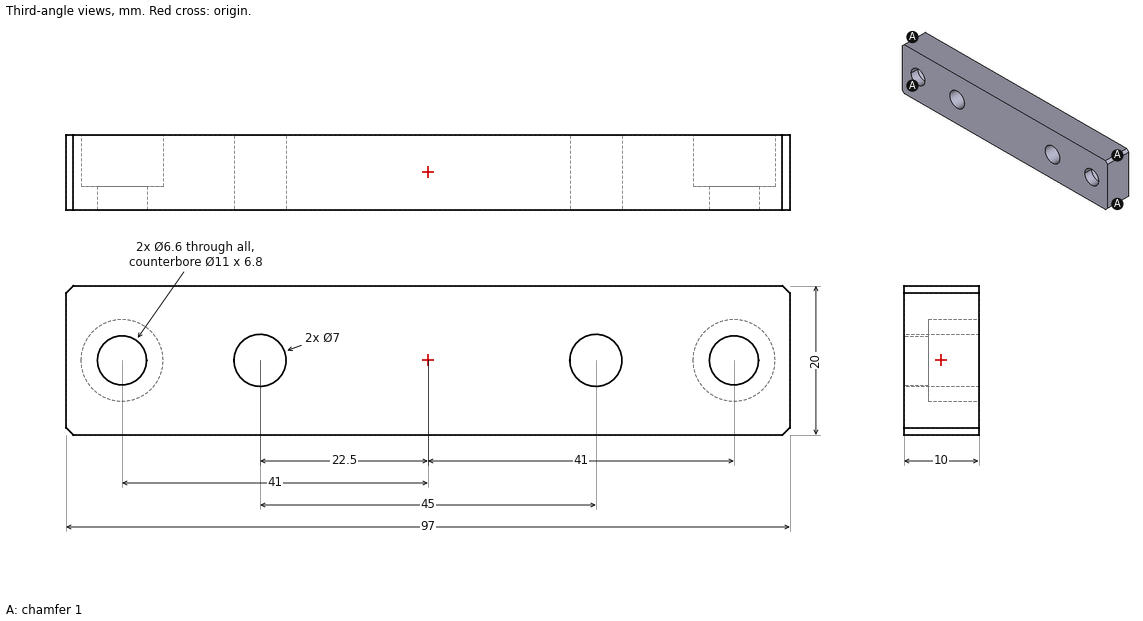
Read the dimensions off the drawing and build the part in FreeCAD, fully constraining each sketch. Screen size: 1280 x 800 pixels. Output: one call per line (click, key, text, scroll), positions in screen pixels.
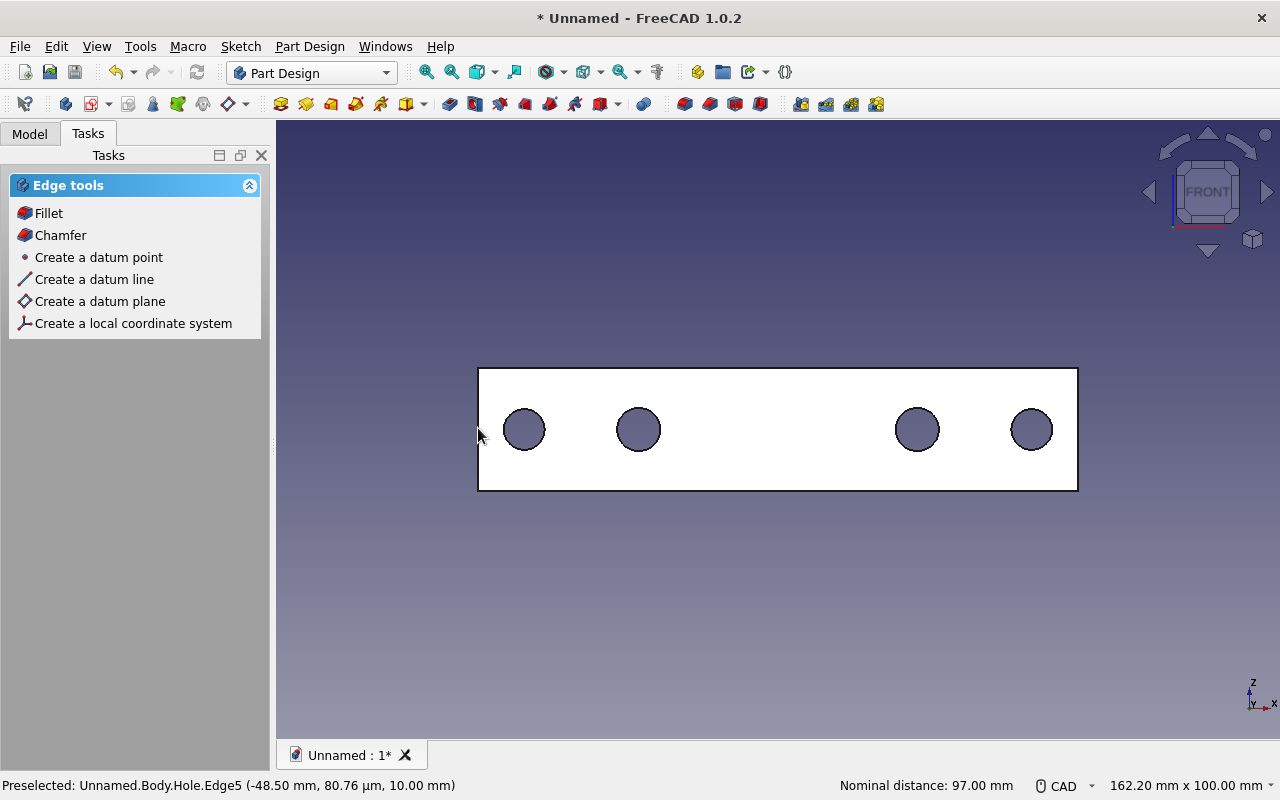
key(3)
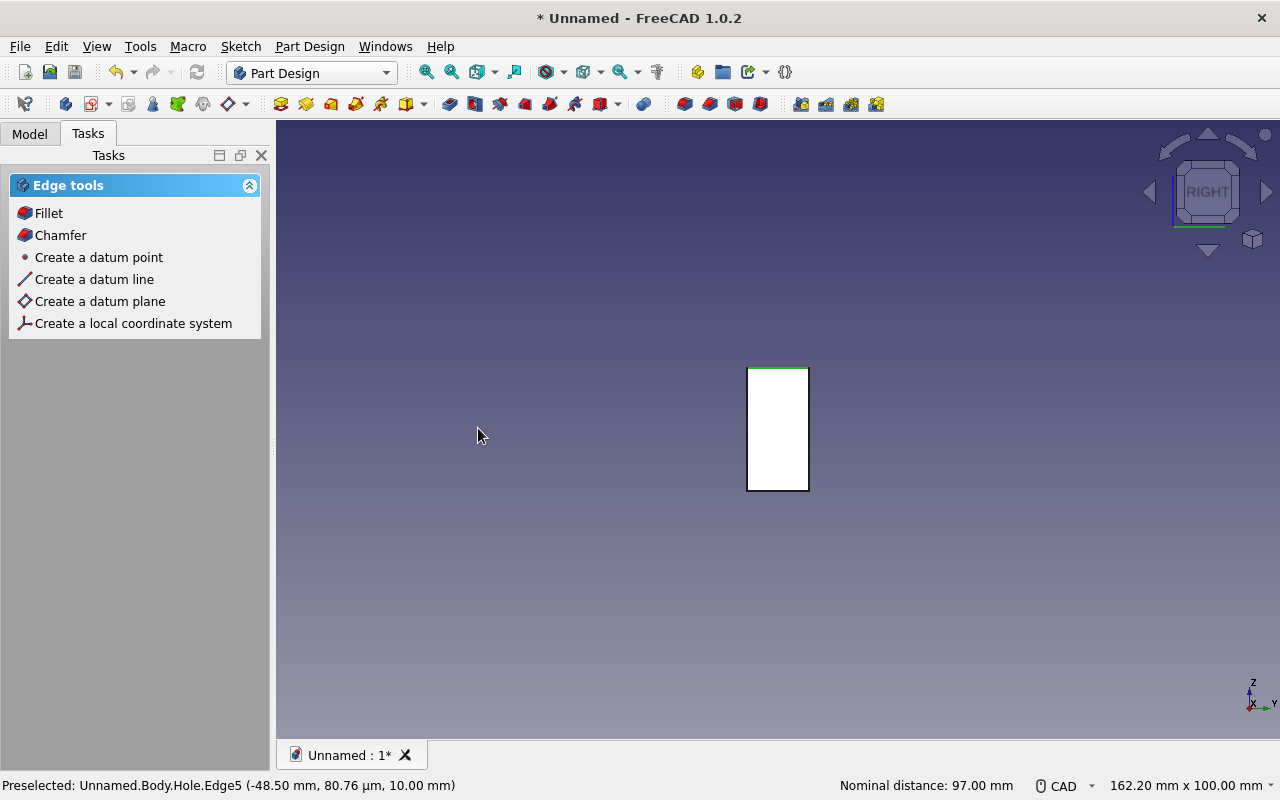
key(v)
key(f)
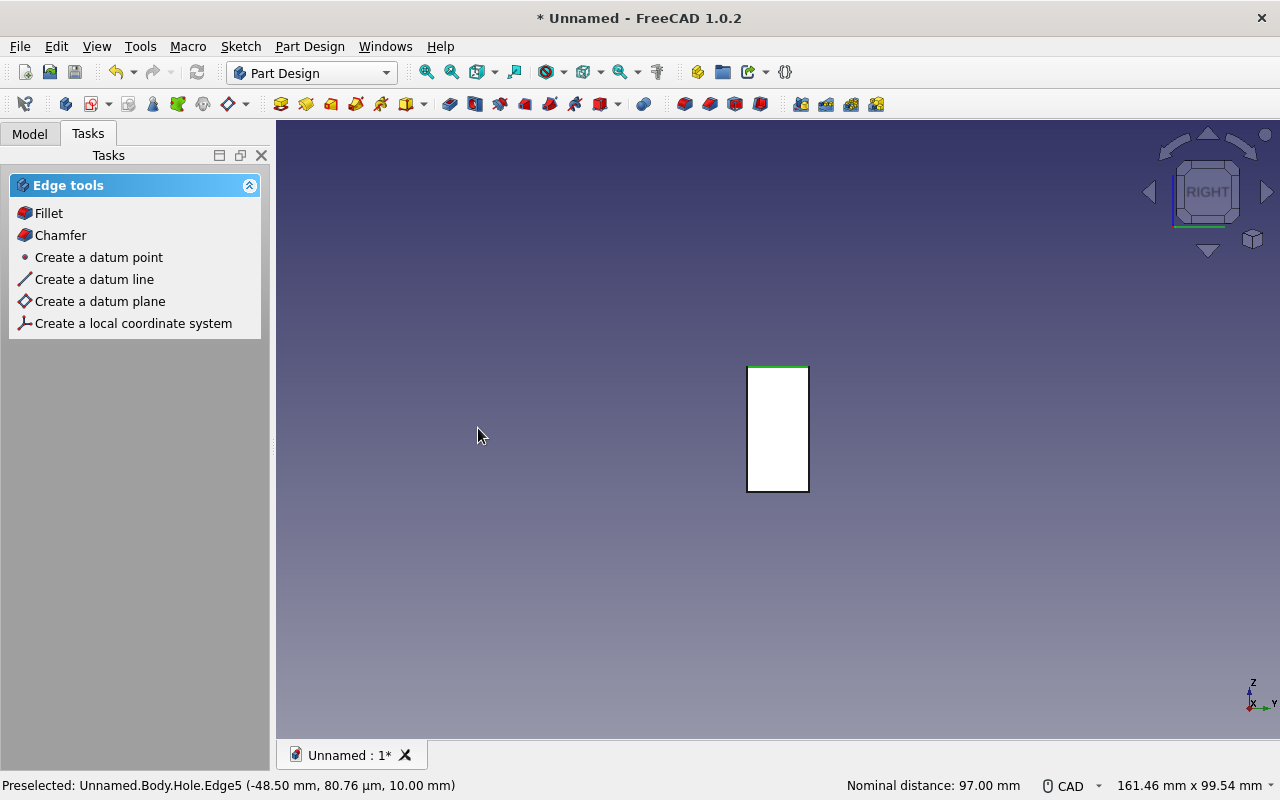
click(778, 491, ctrl)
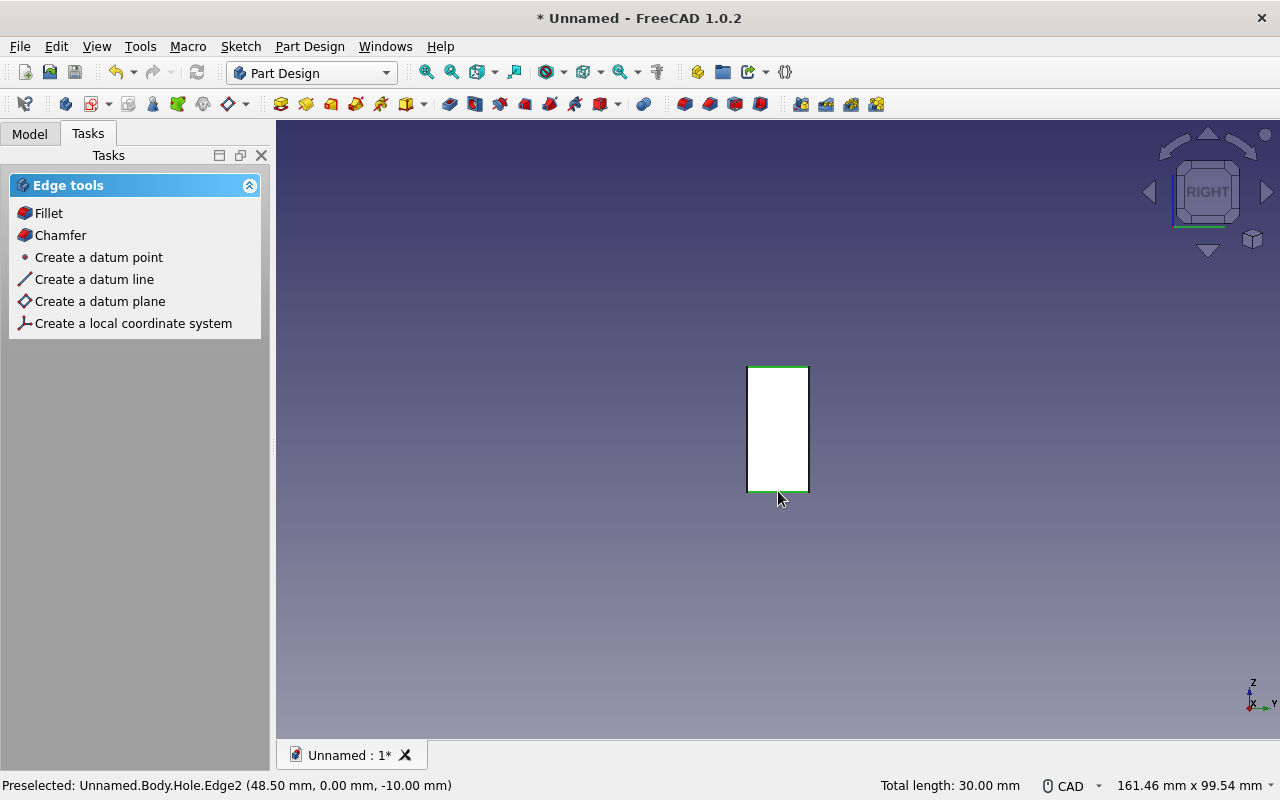
key(5)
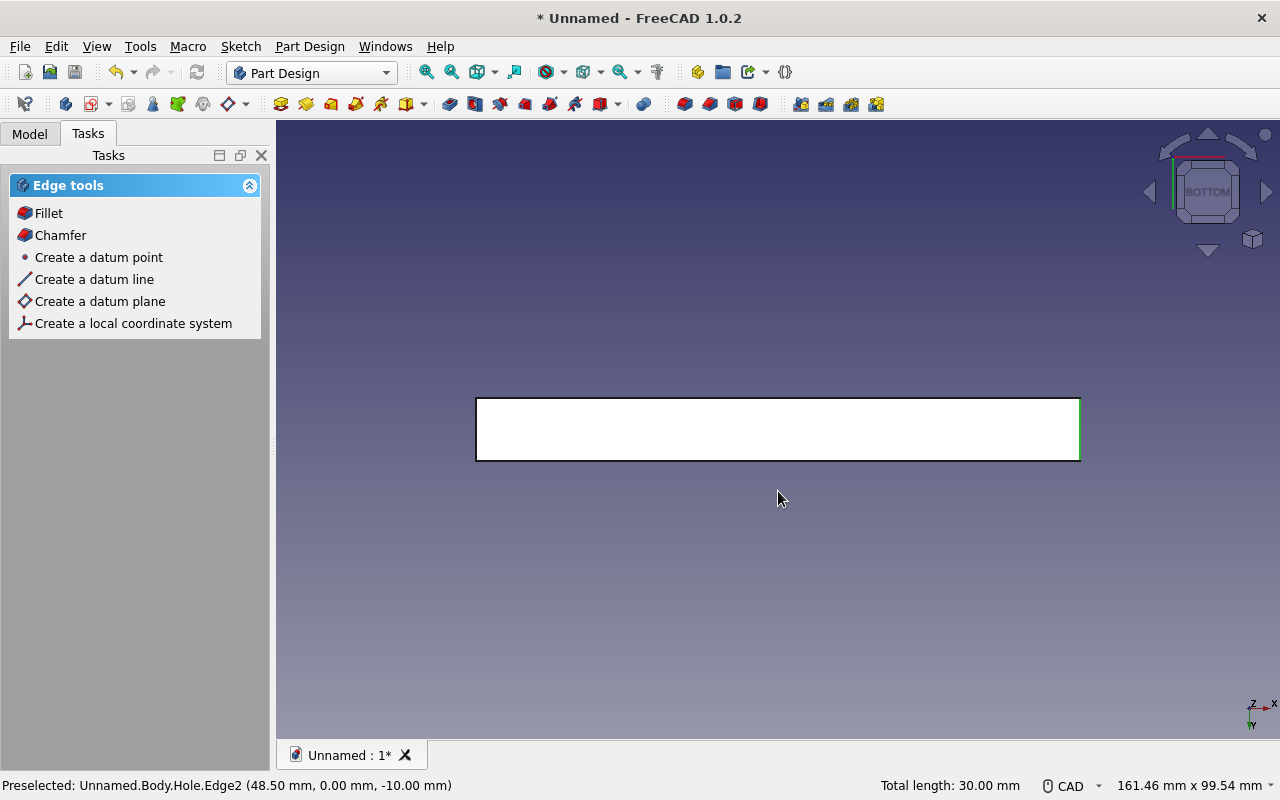
click(476, 428, ctrl)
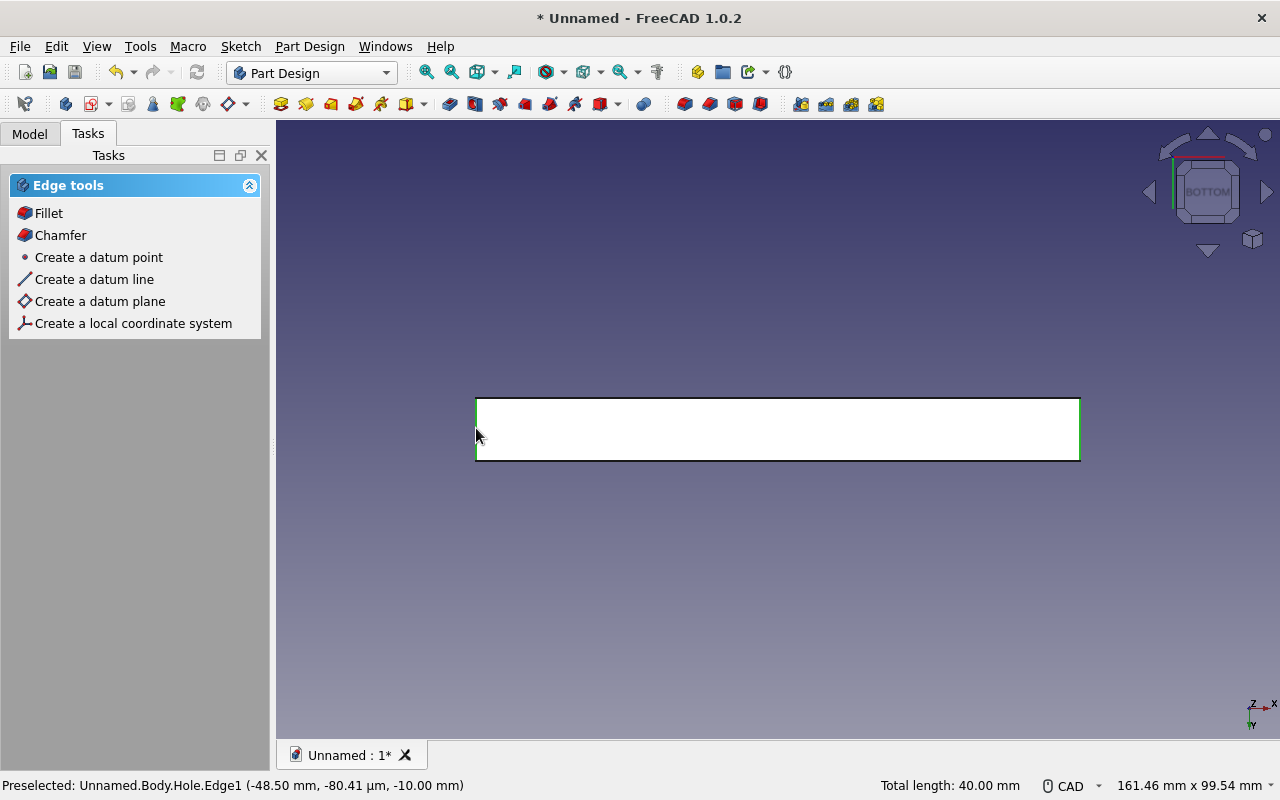
click(710, 104)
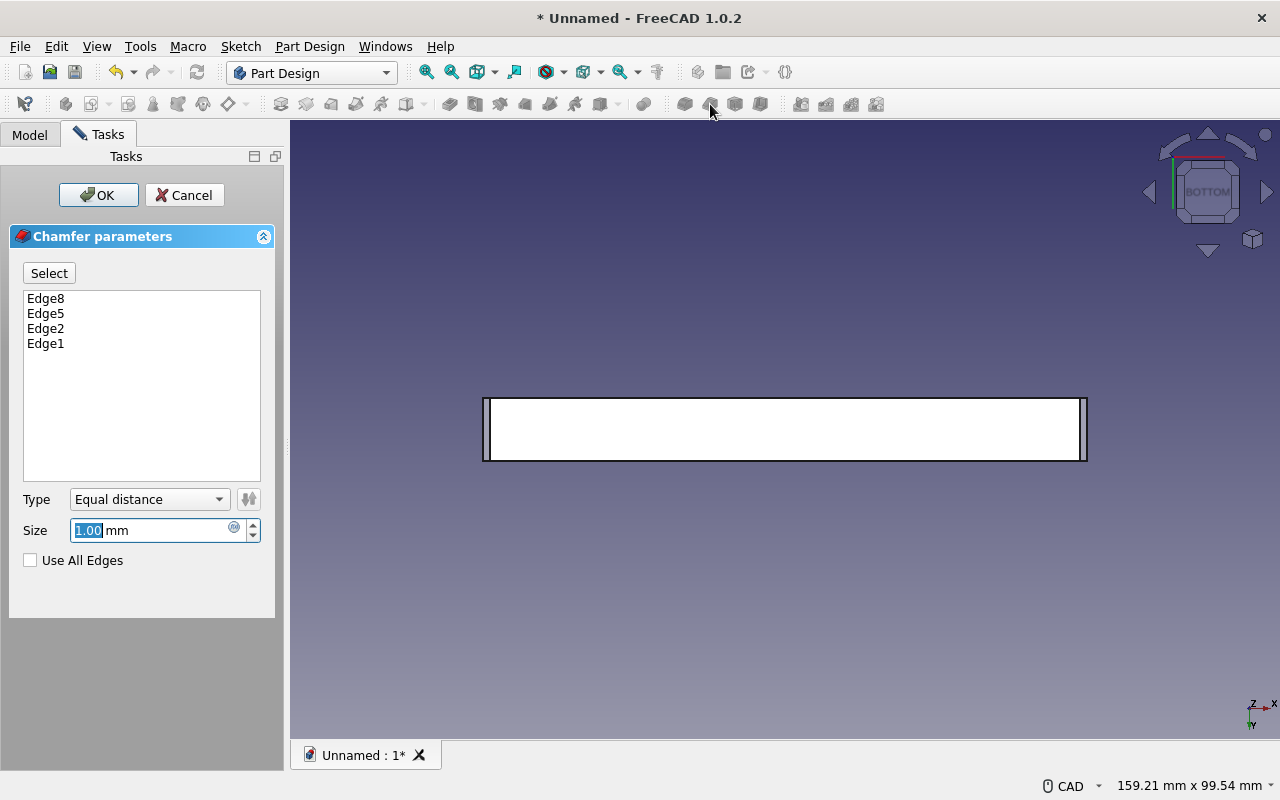
text(1)
key(Tab)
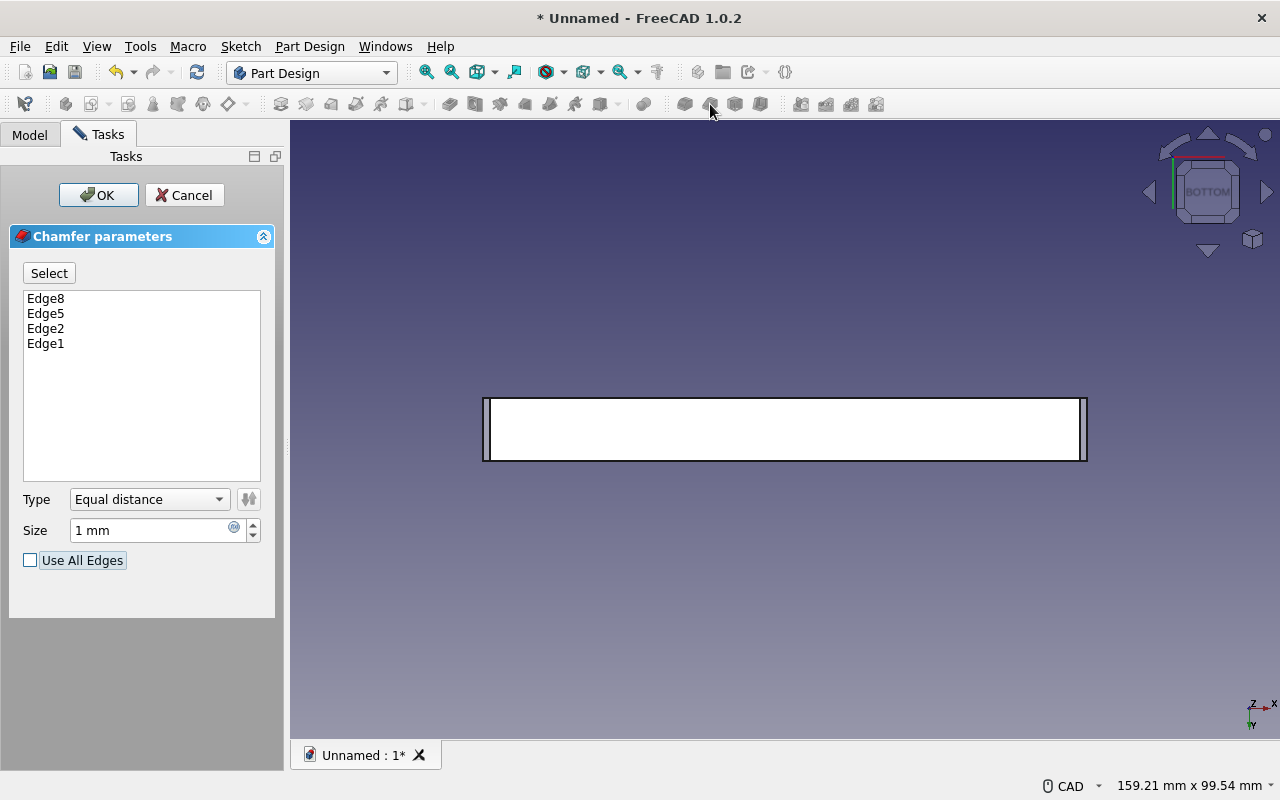
click(99, 195)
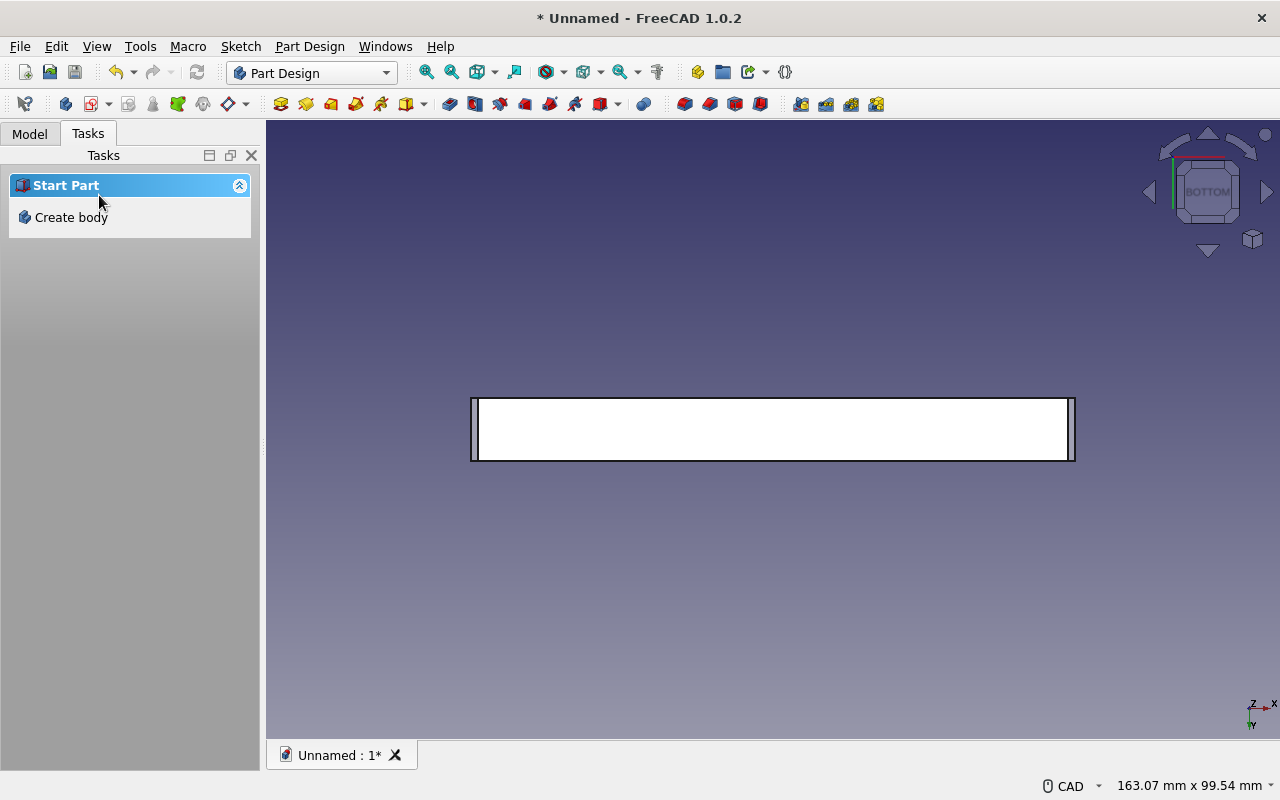
key(0)